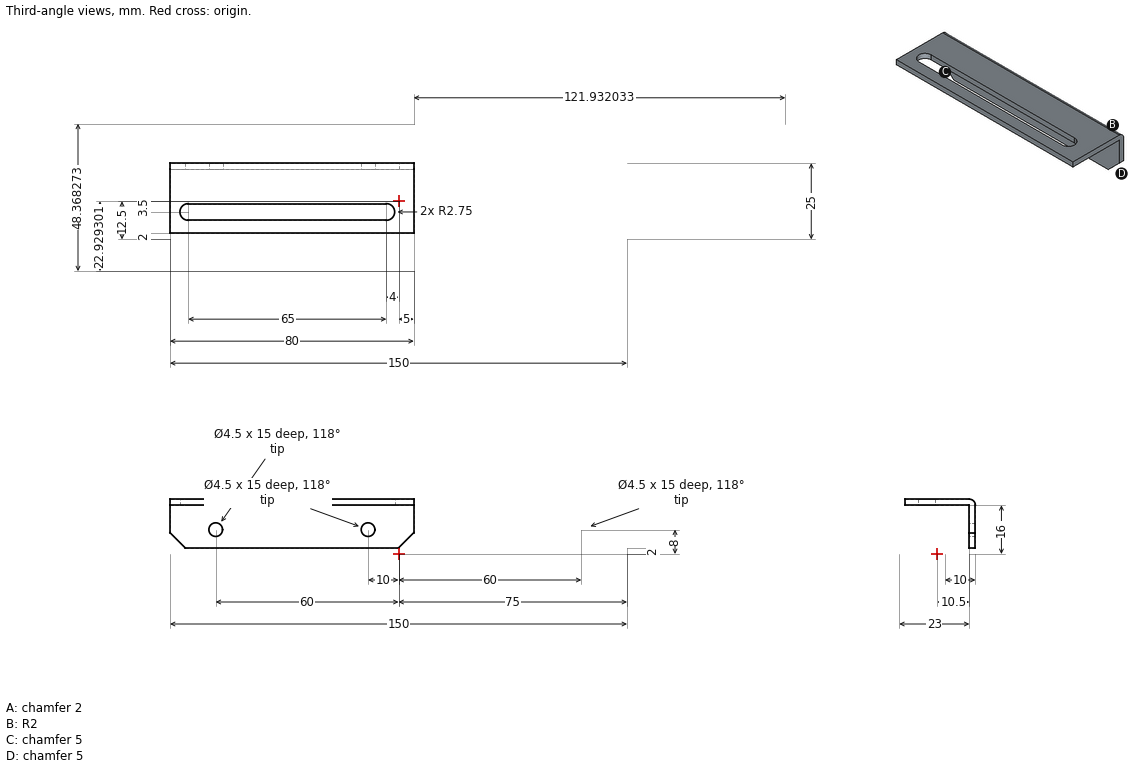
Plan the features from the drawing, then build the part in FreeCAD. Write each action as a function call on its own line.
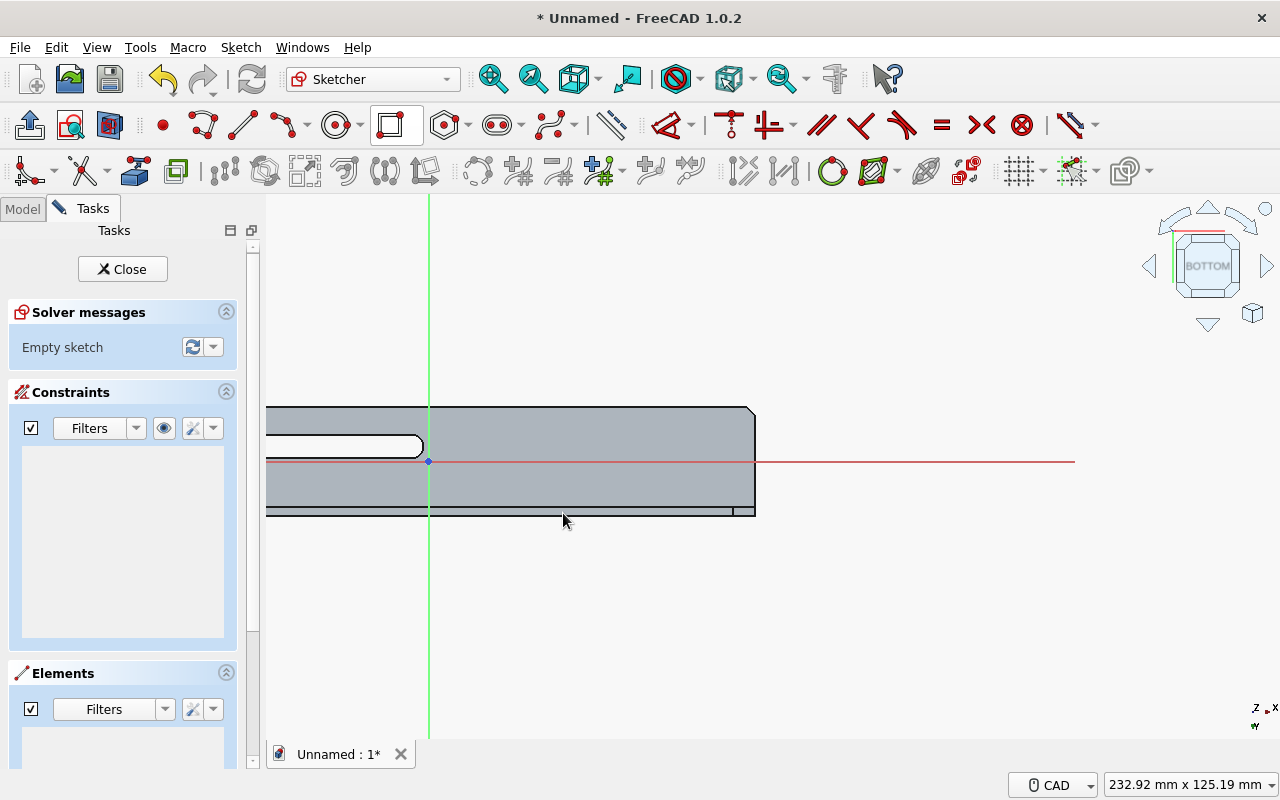
click(390, 126)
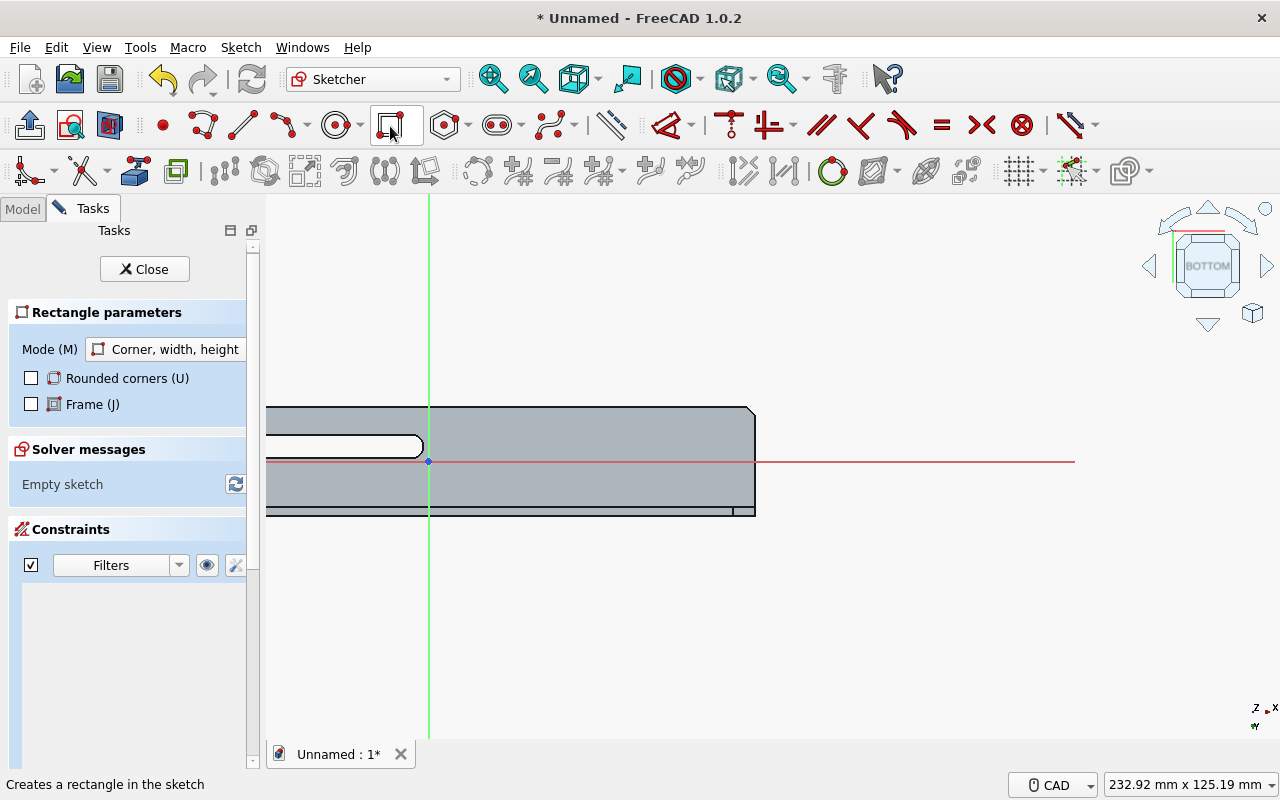
click(450, 362)
click(981, 572)
key(Escape)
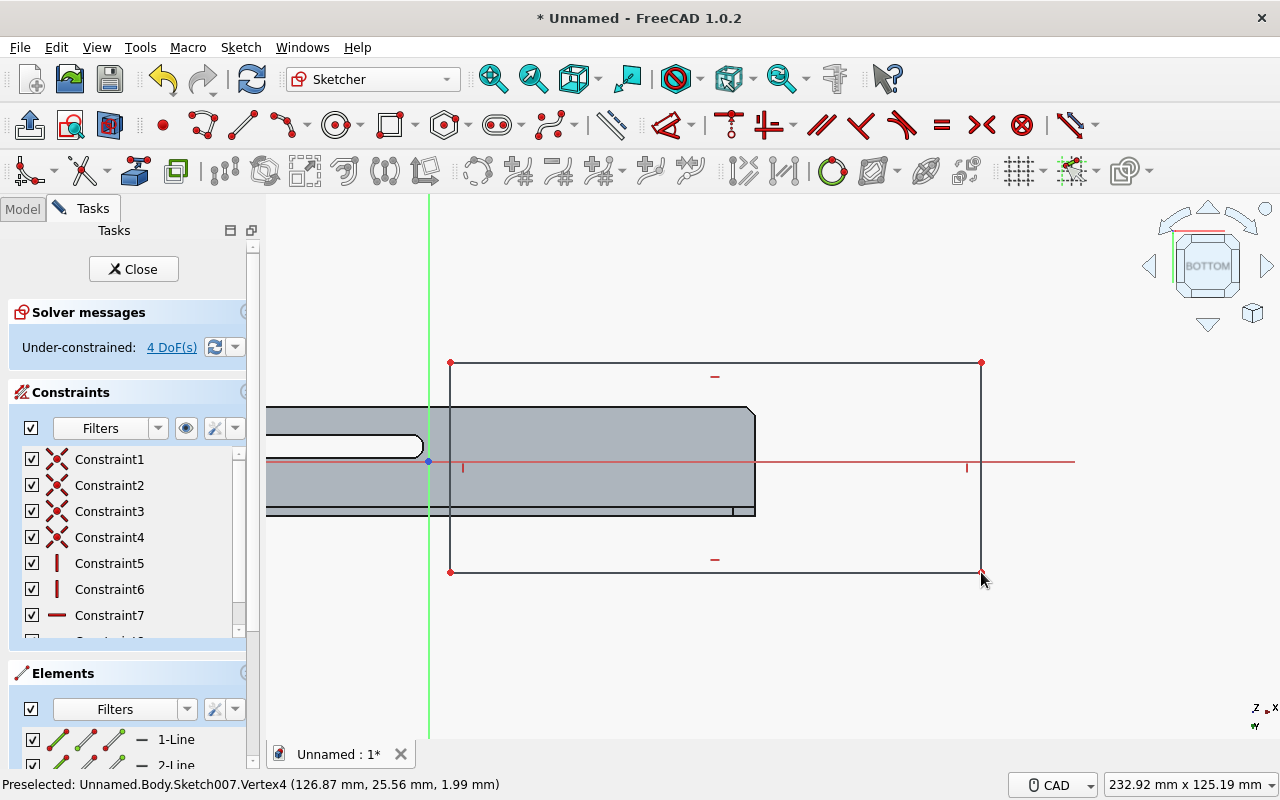
click(666, 126)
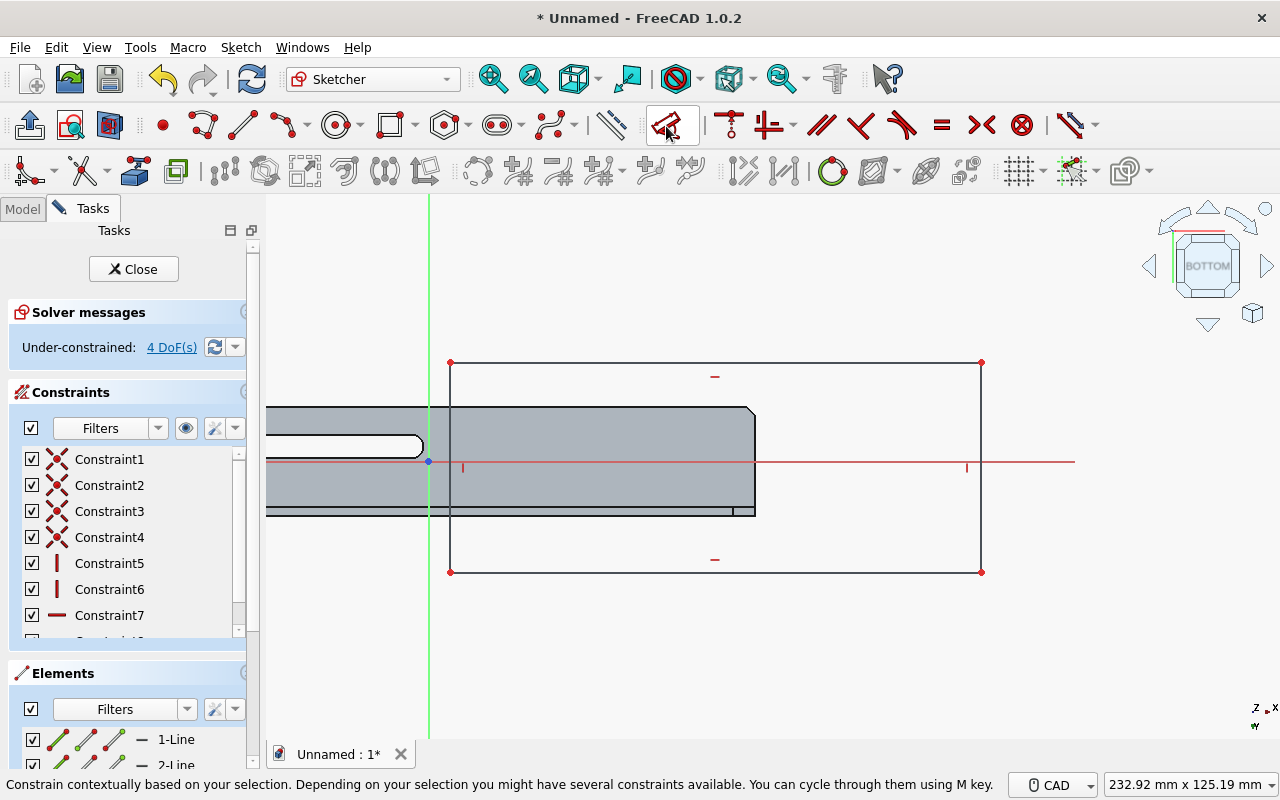
scroll(450, 363, up, 4)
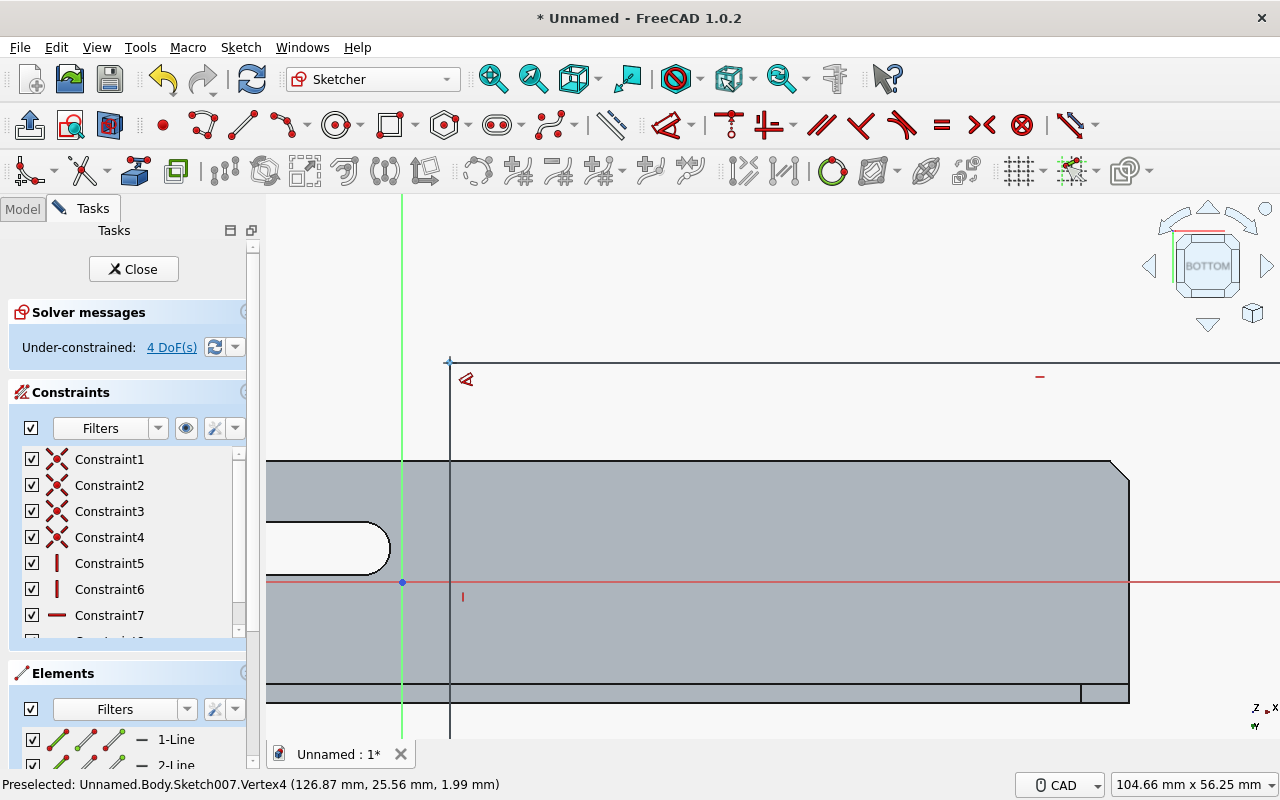
click(450, 363)
click(426, 329)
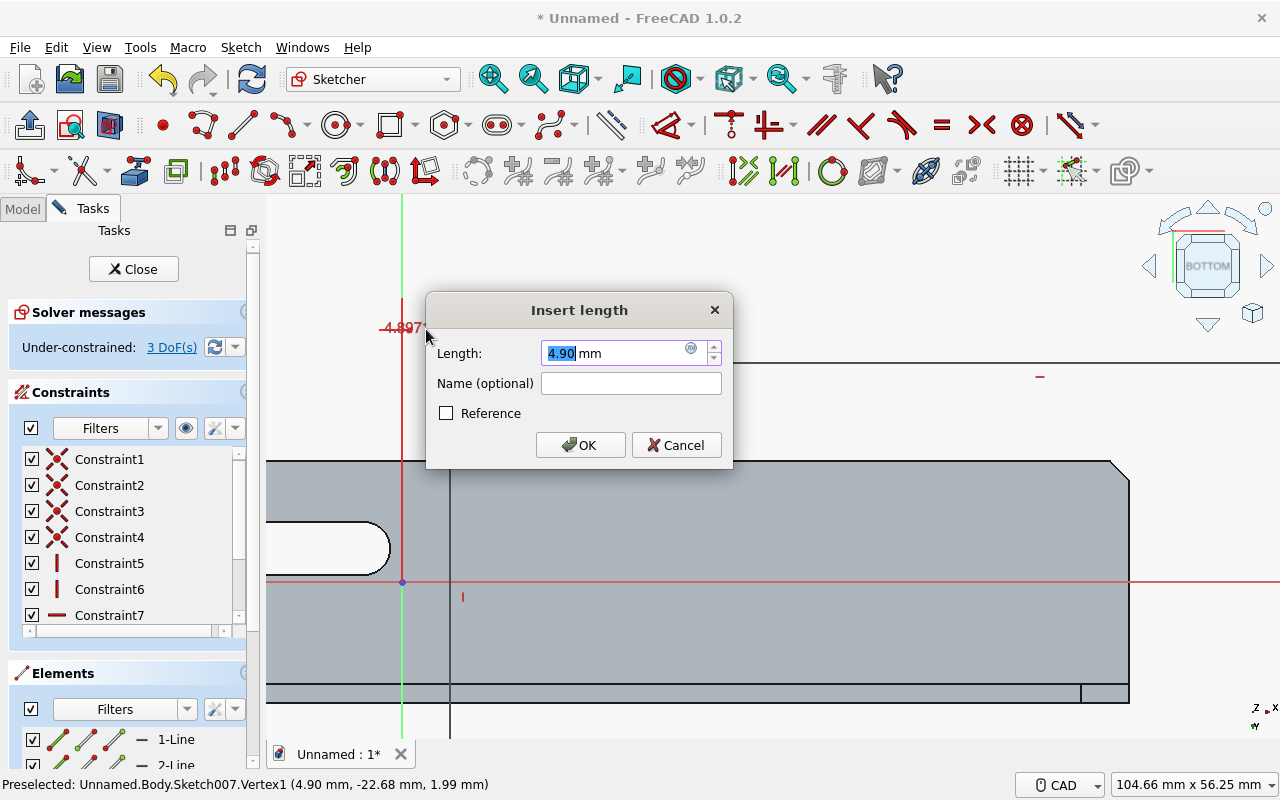
text(5)
key(Return)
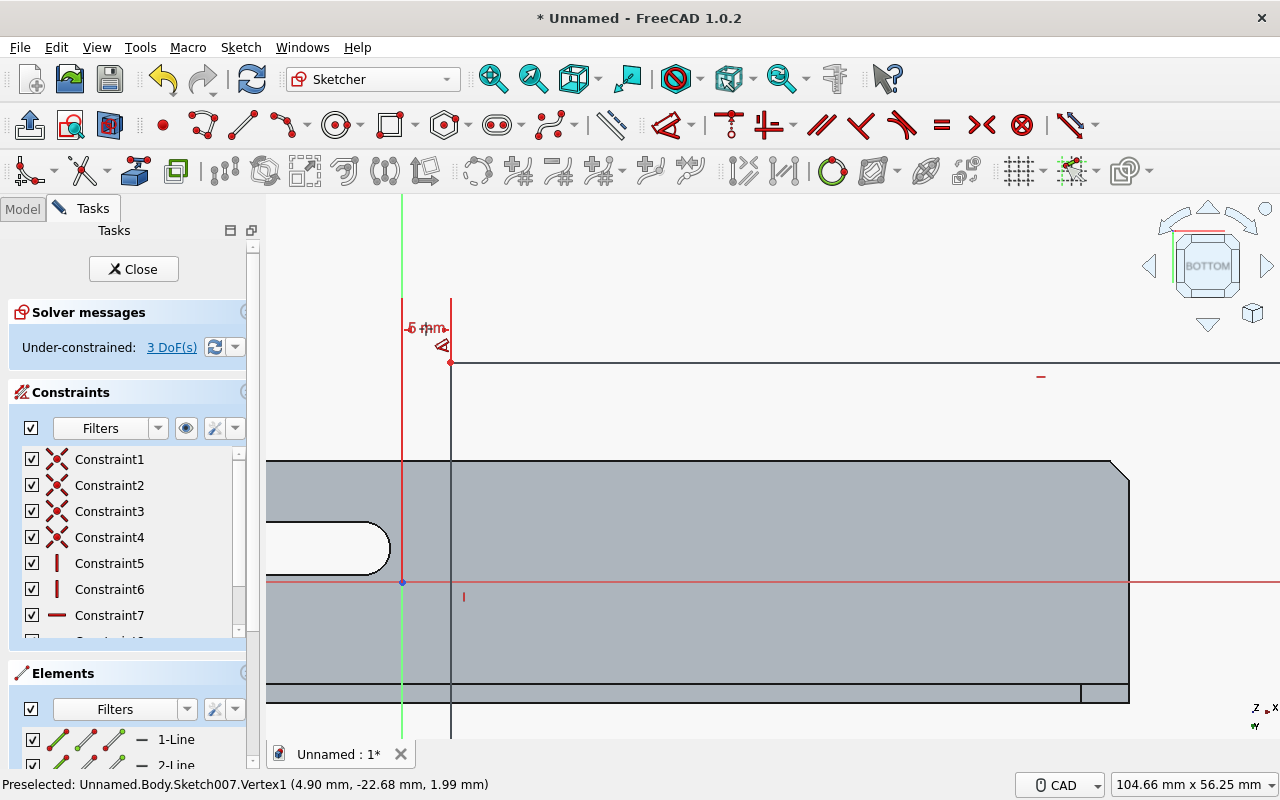
click(451, 503)
click(417, 537)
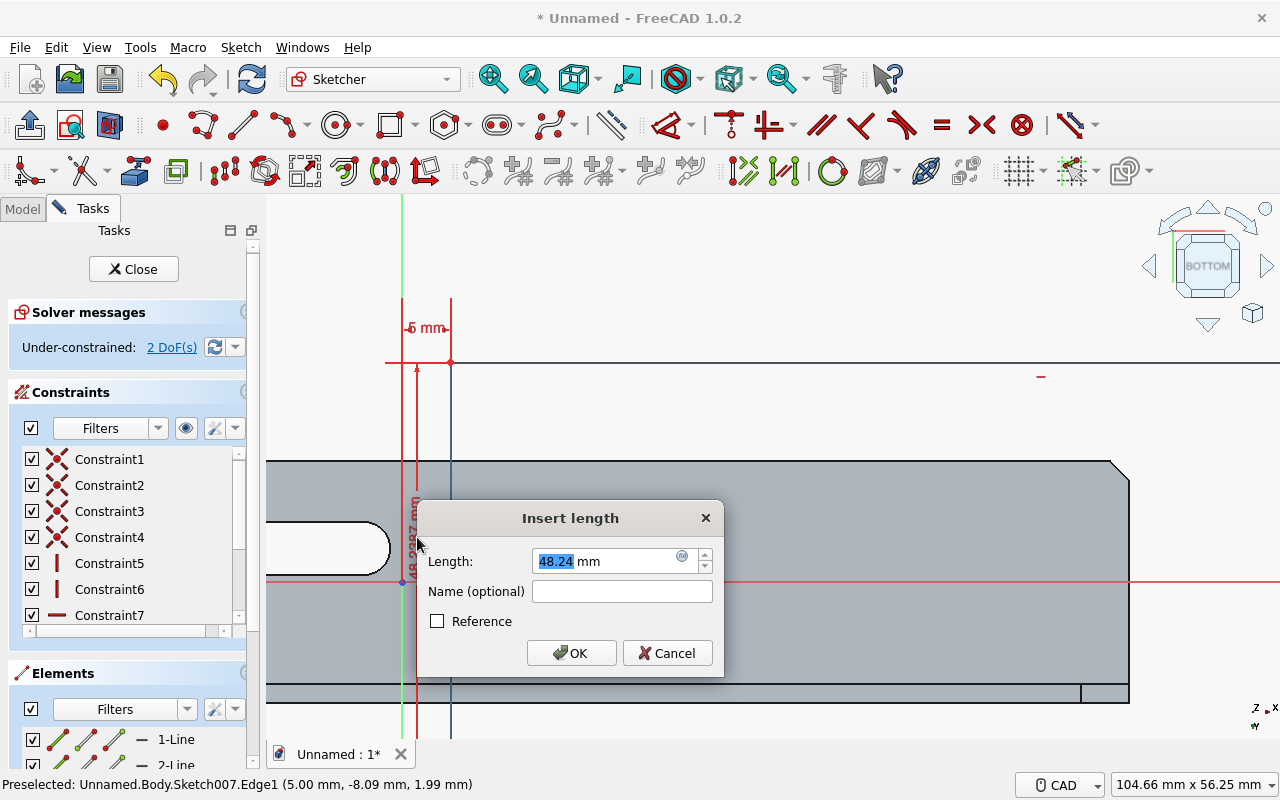
text(48.368273)
key(Return)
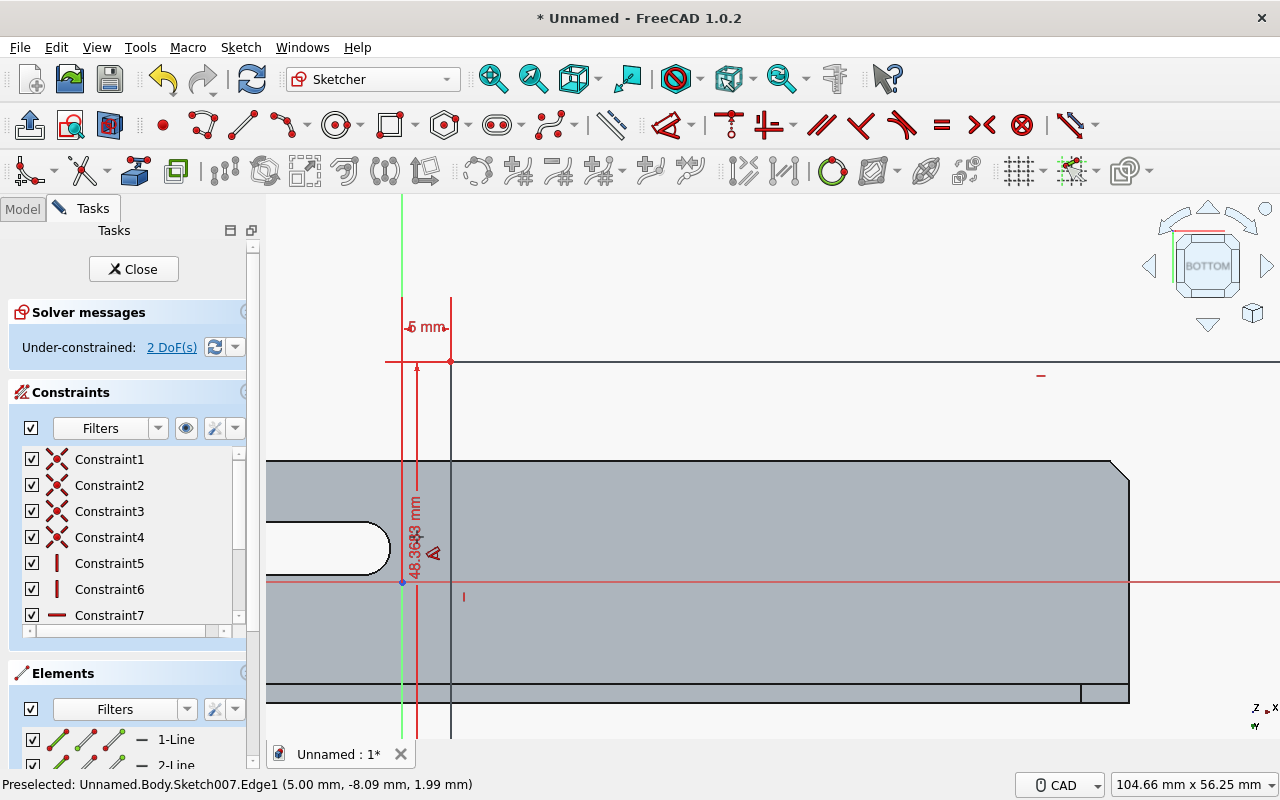
scroll(449, 362, down, 4)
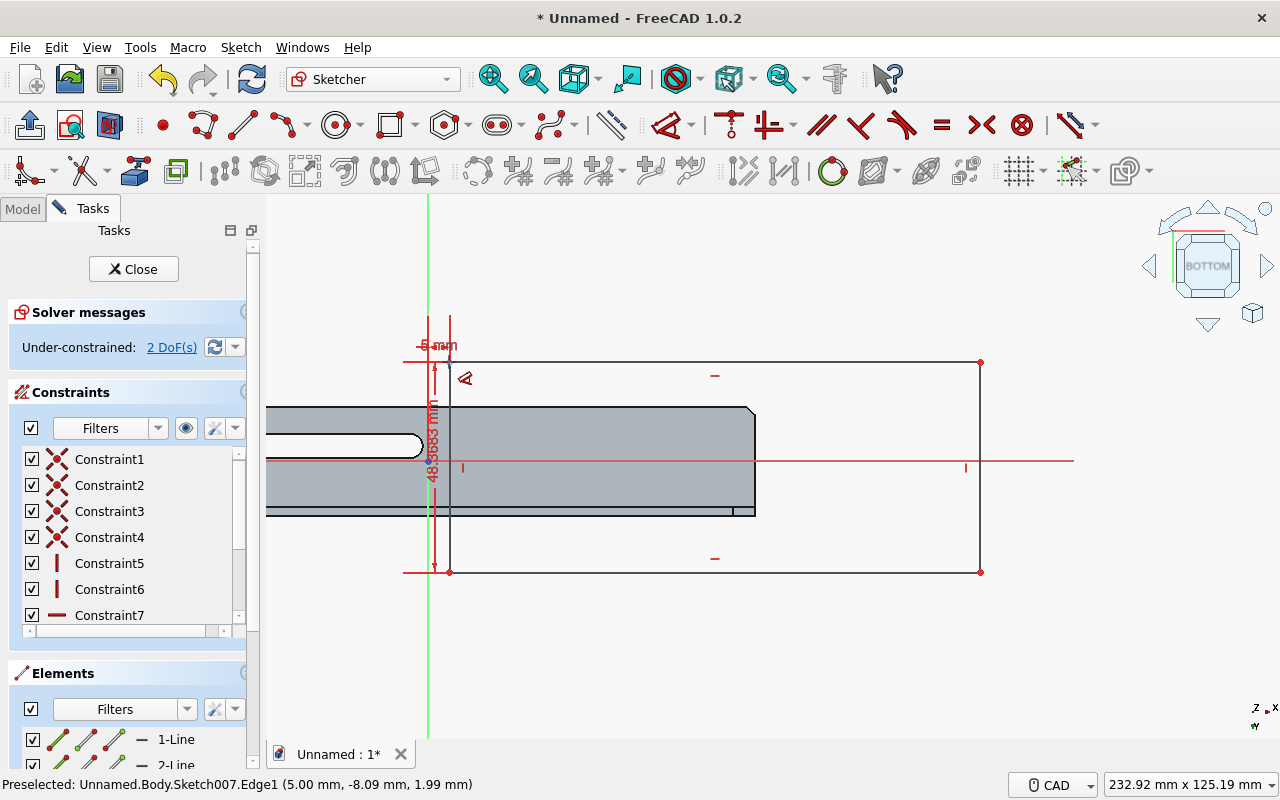
click(609, 573)
click(715, 607)